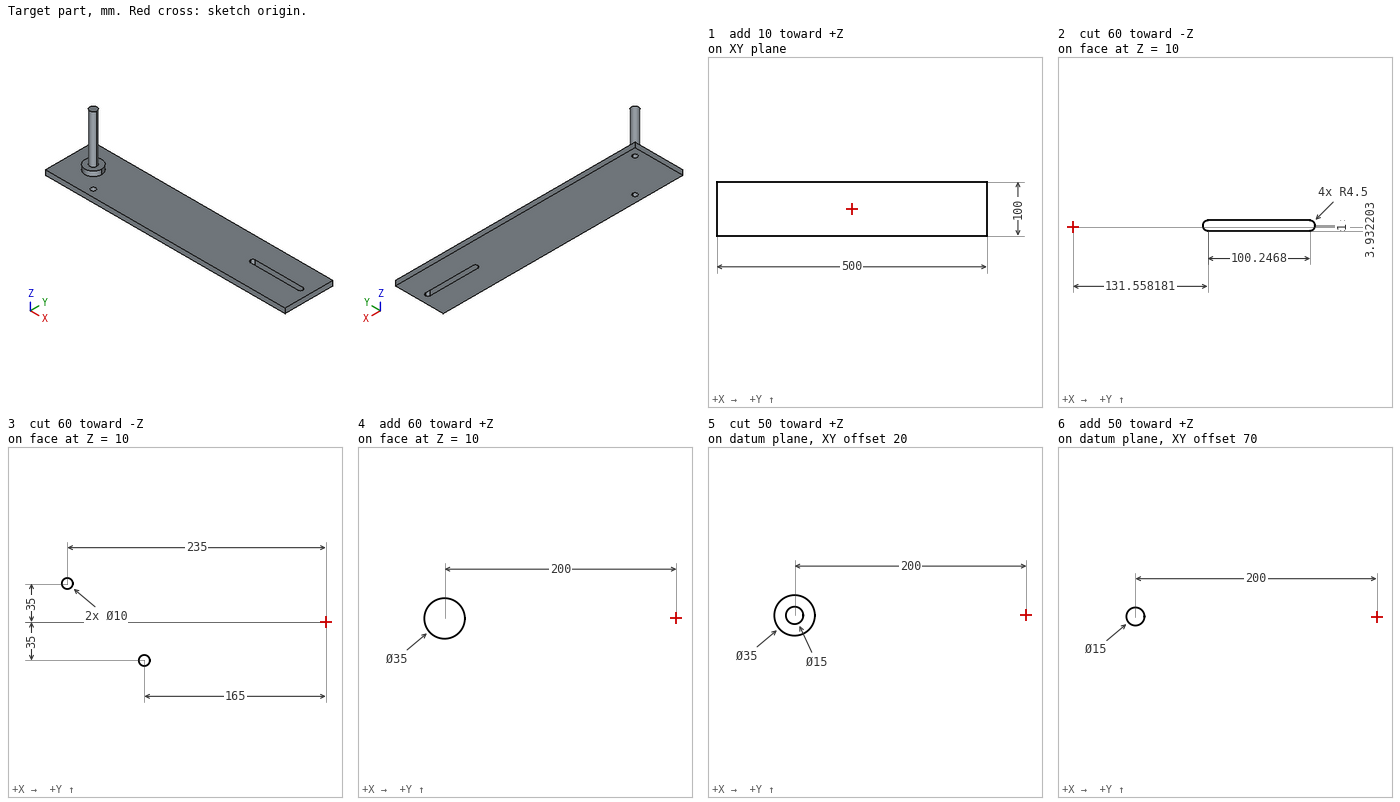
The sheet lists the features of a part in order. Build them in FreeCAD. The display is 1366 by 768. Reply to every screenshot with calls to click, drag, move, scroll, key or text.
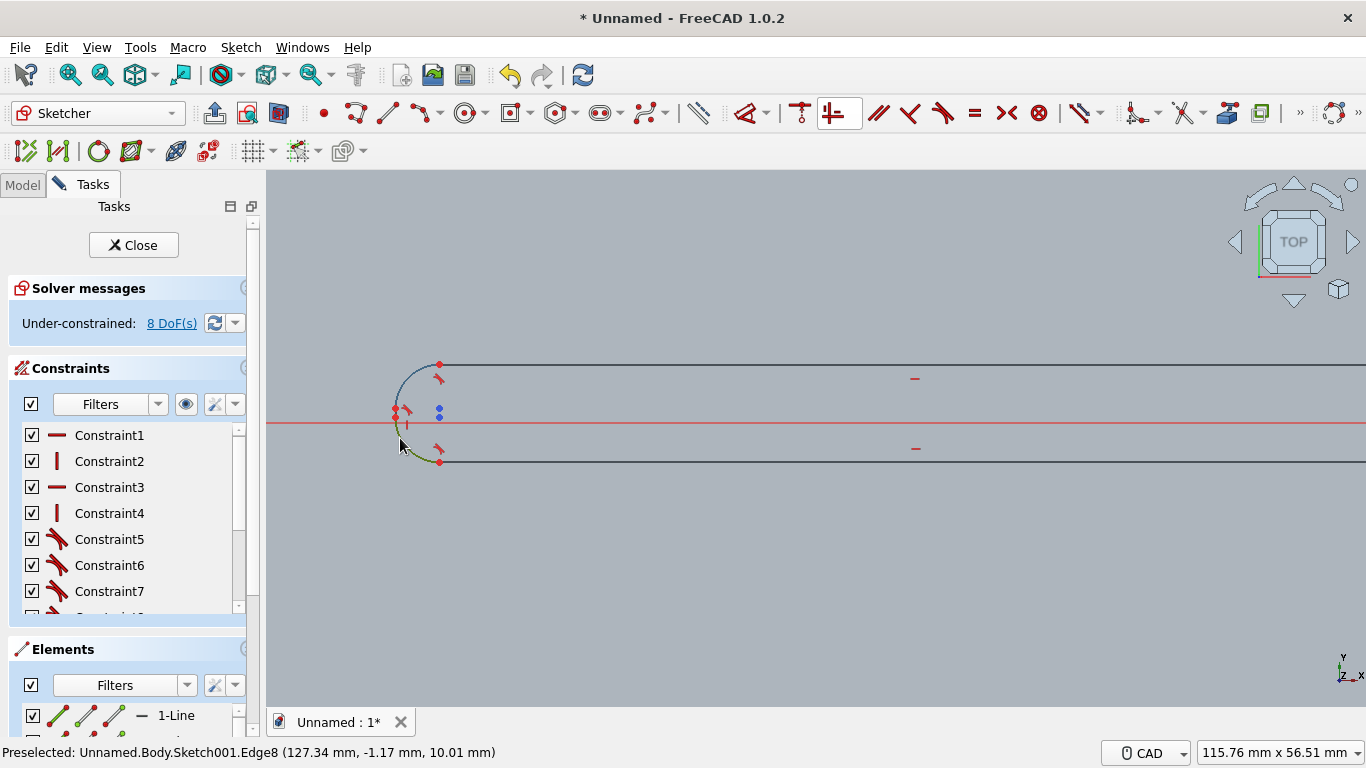
key(e)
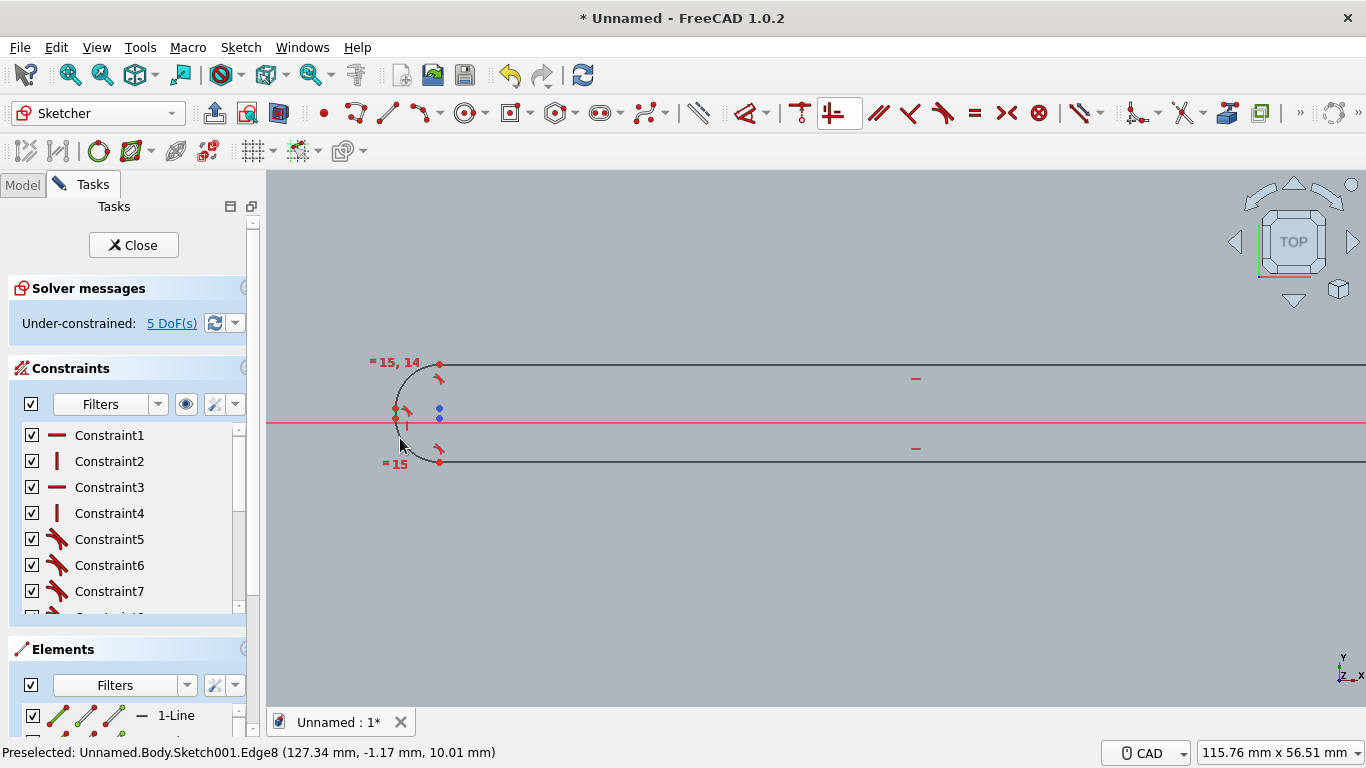
key(d)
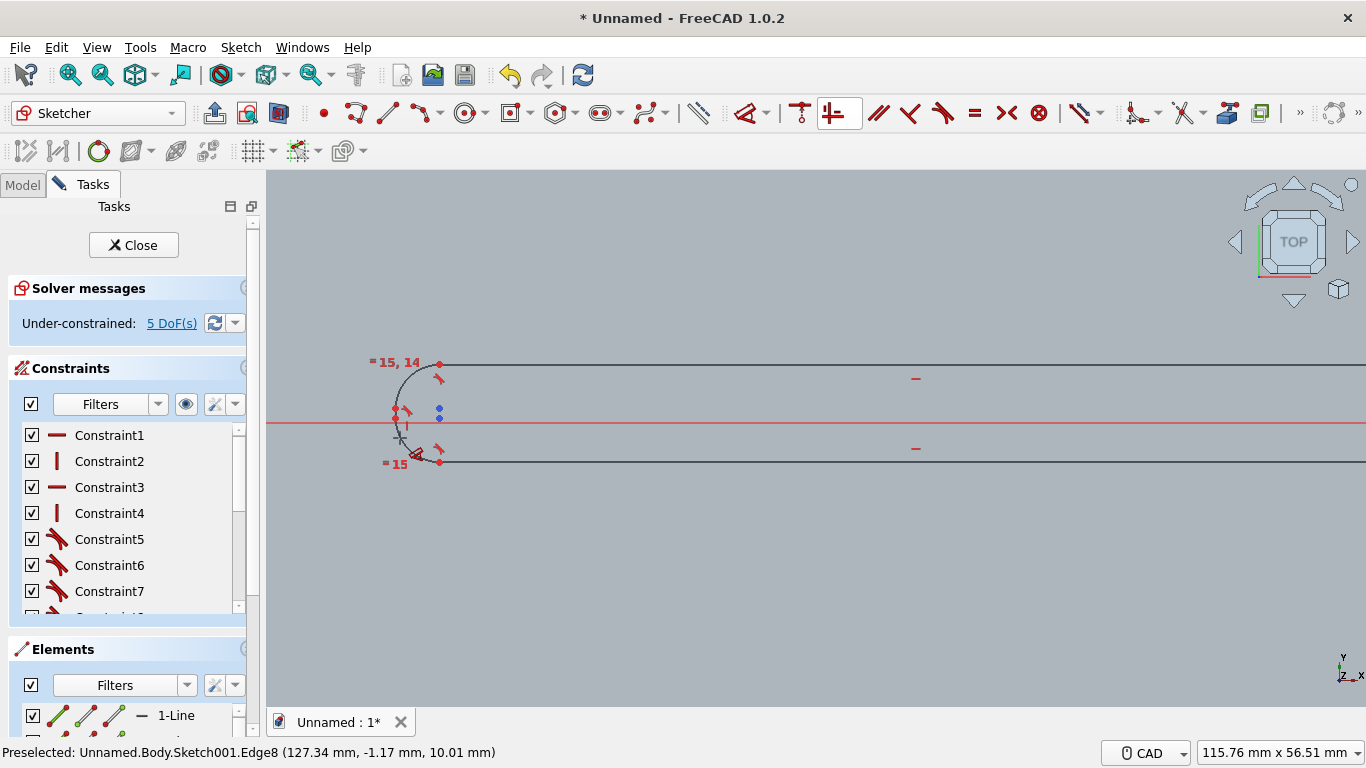
scroll(935, 449, down, 6)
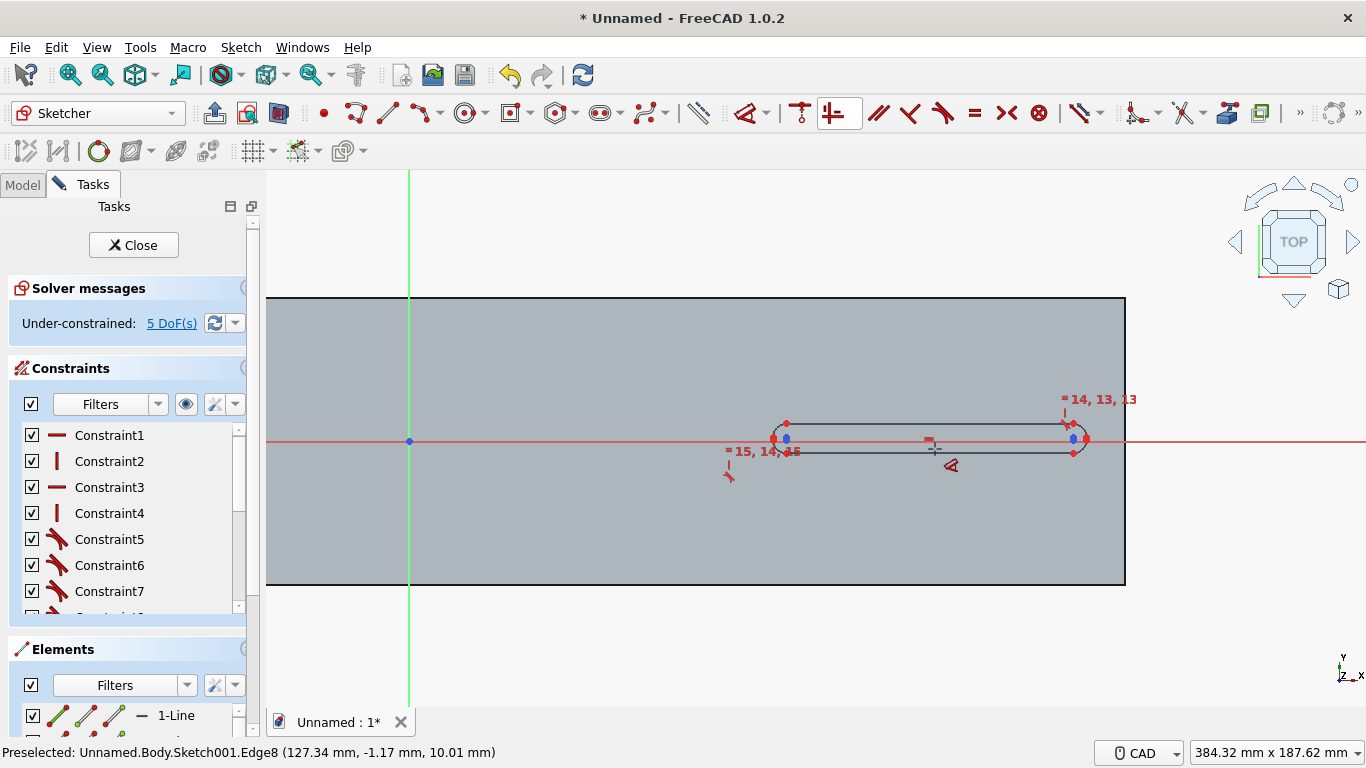
scroll(1079, 452, up, 6)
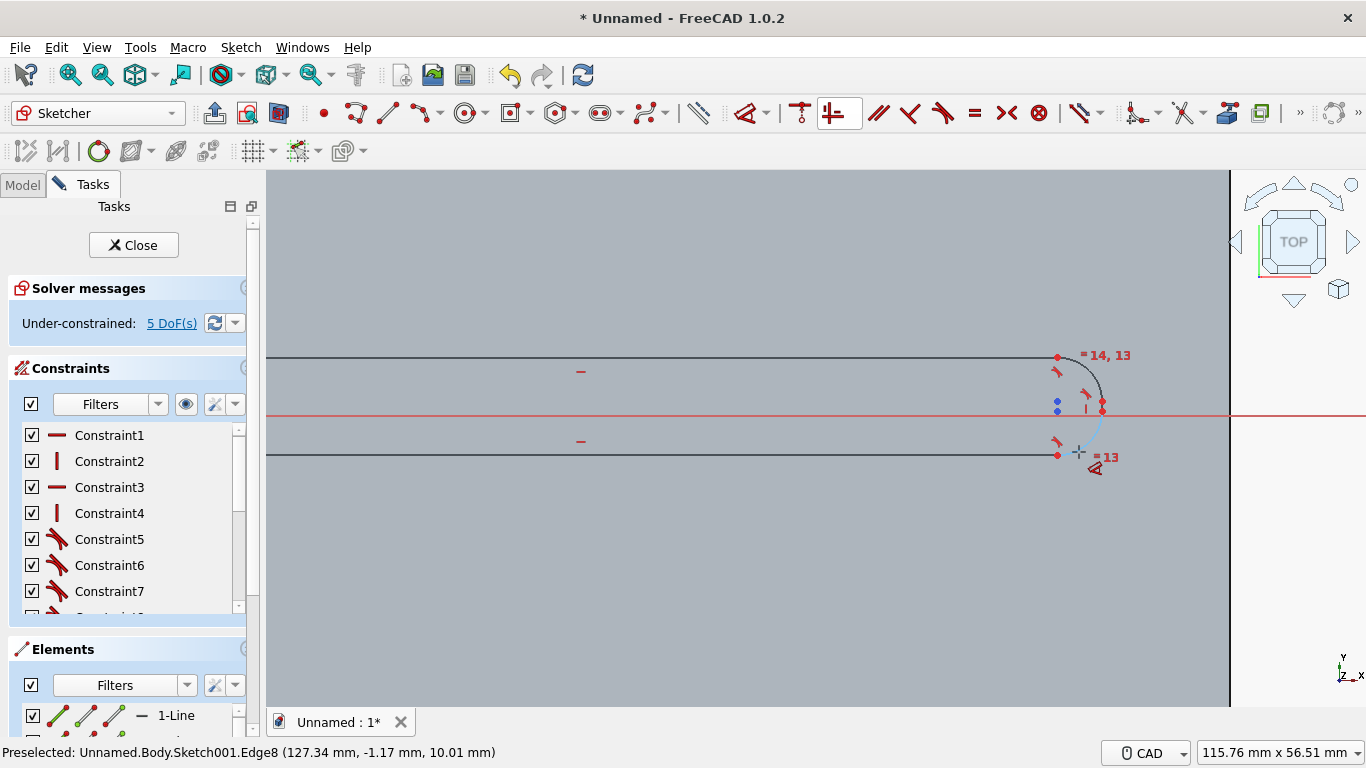
click(1078, 451)
click(1092, 480)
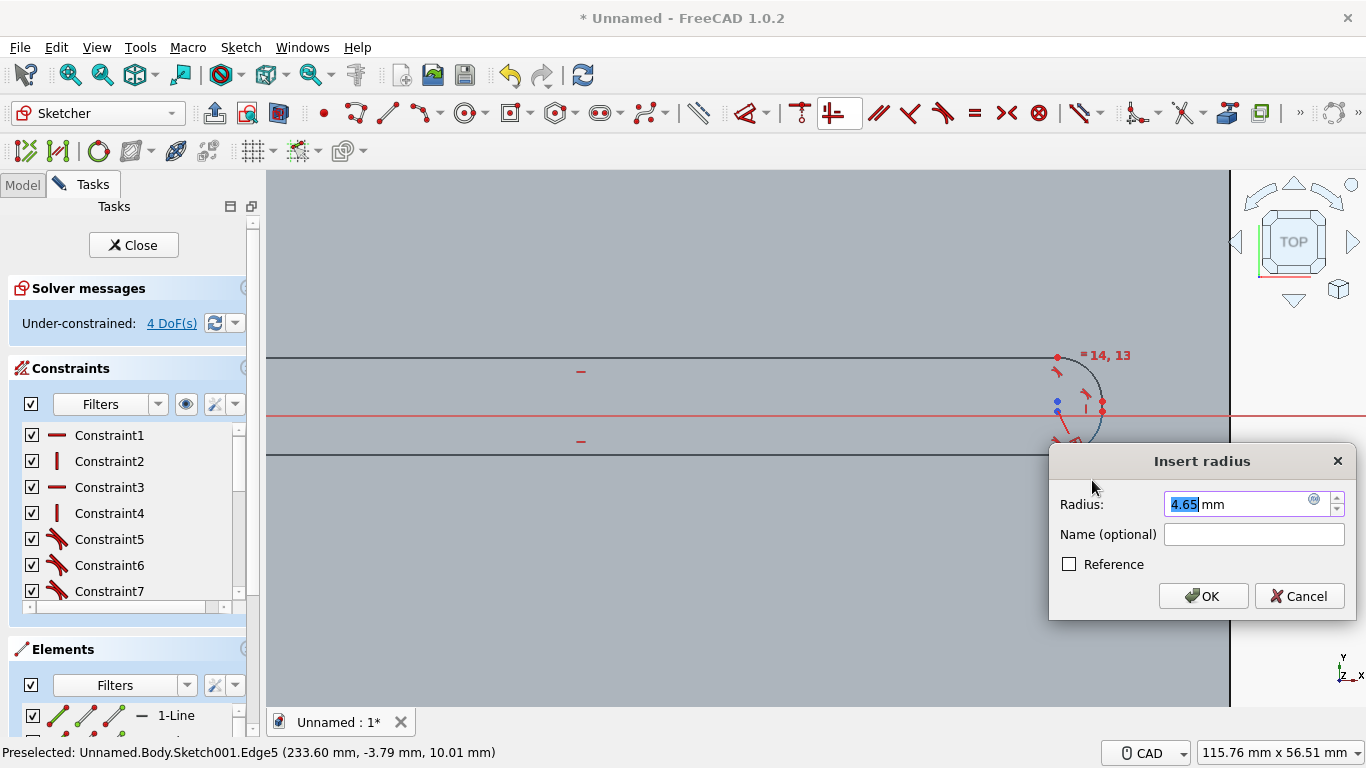
text(4.5)
key(Return)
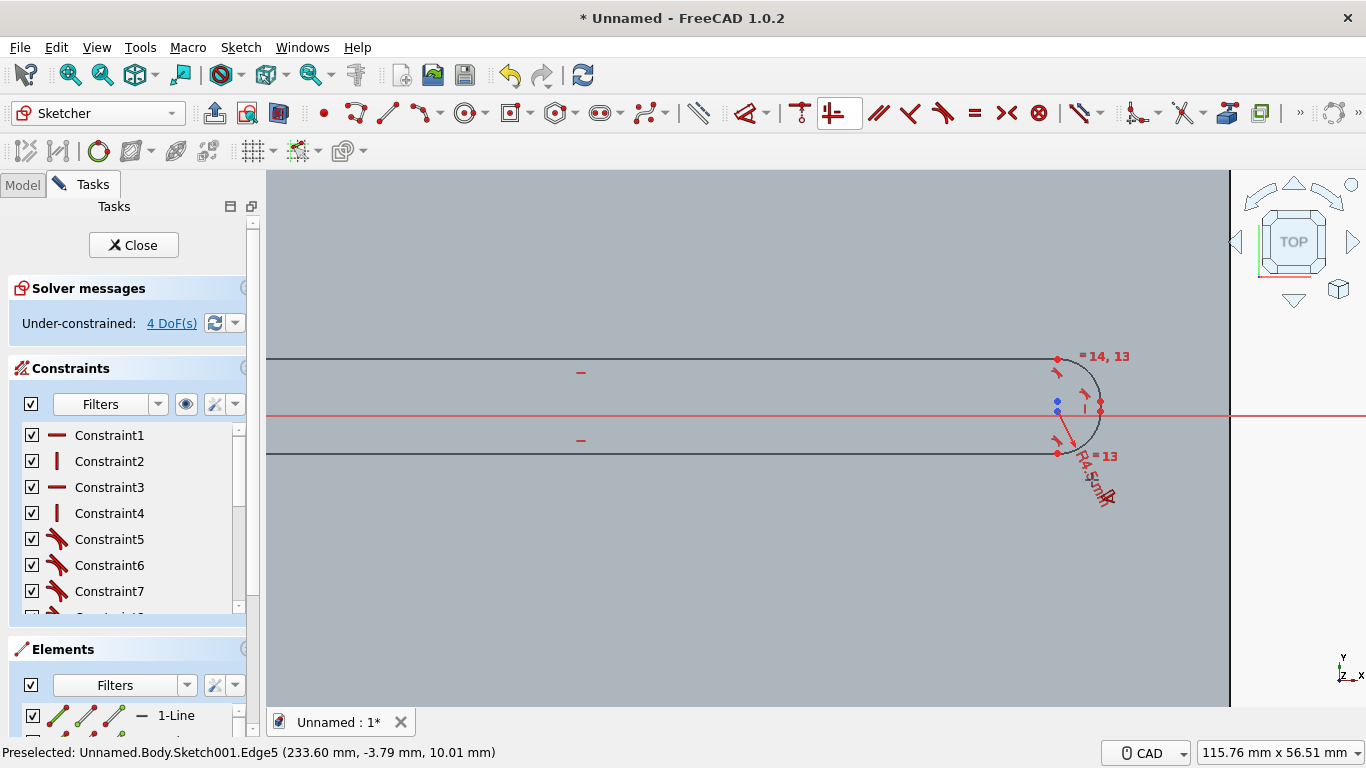
scroll(1101, 407, up, 8)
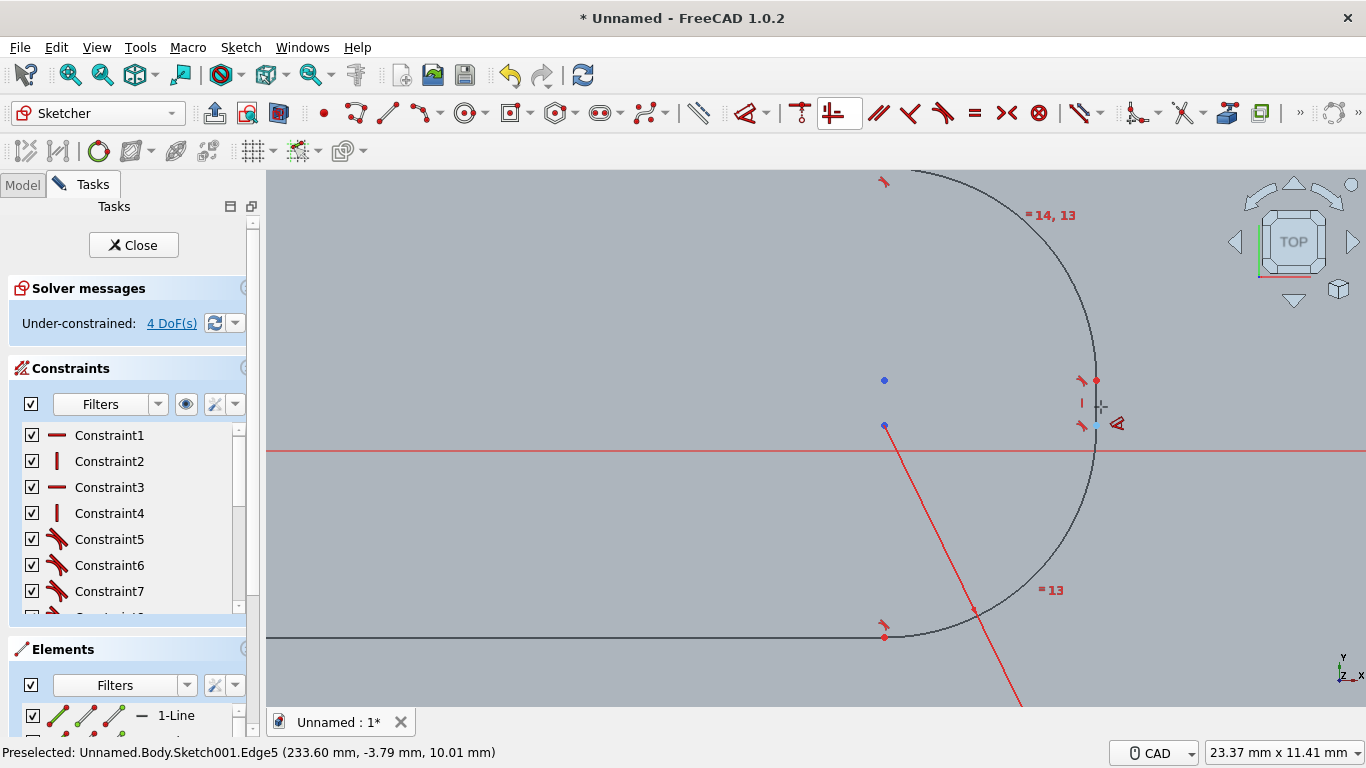
click(1096, 403)
click(1130, 403)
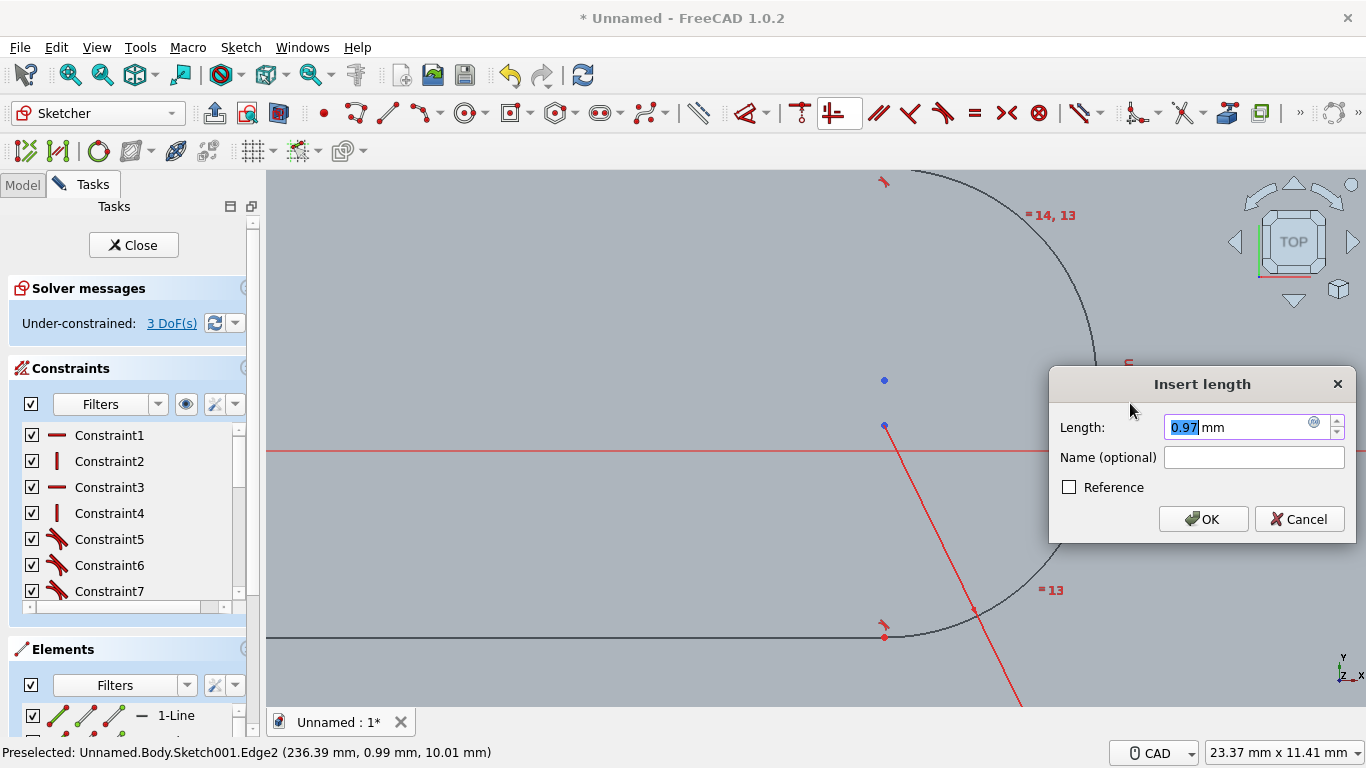
text(1)
key(Return)